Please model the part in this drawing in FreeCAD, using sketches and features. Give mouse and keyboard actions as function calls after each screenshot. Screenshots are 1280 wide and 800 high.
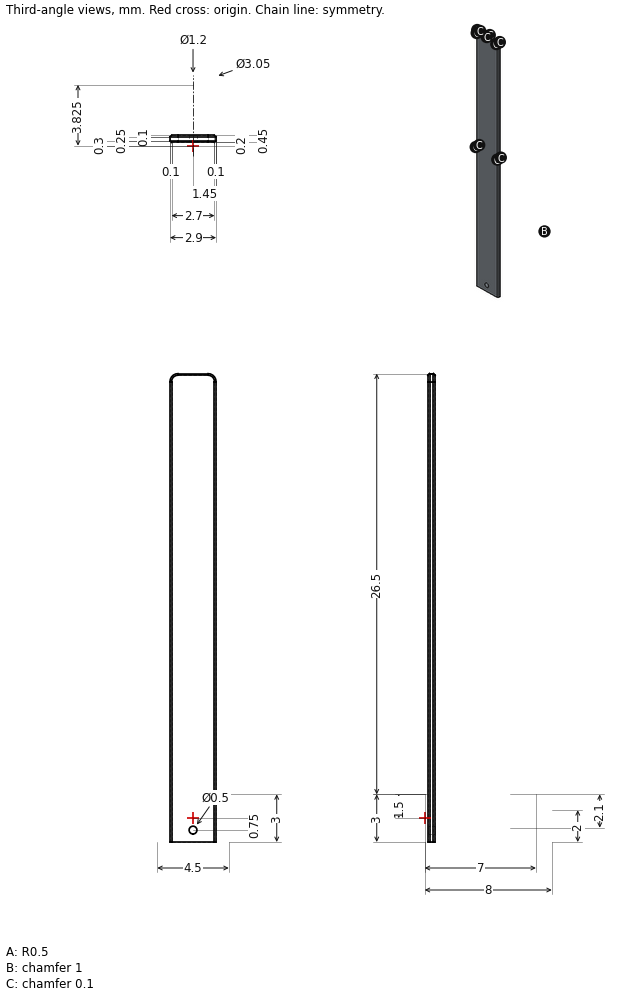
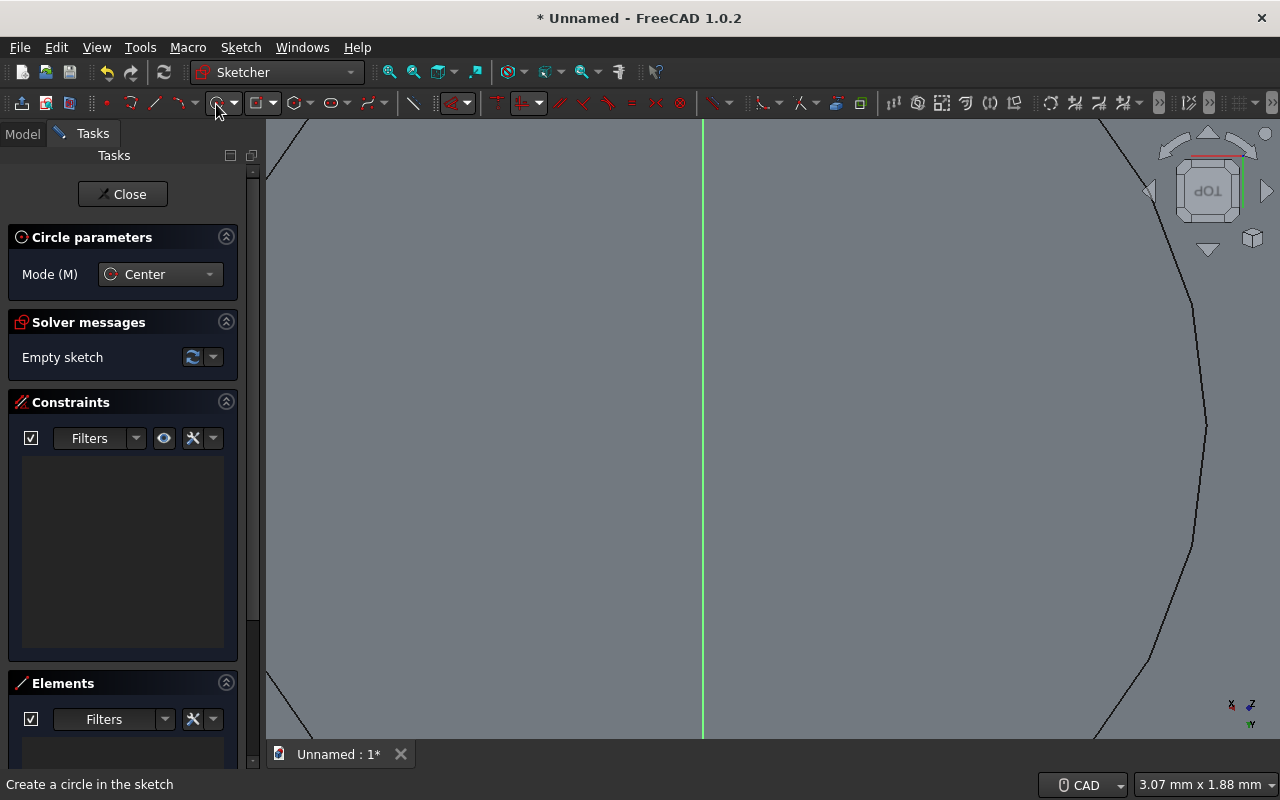
click(703, 425)
click(843, 285)
key(Escape)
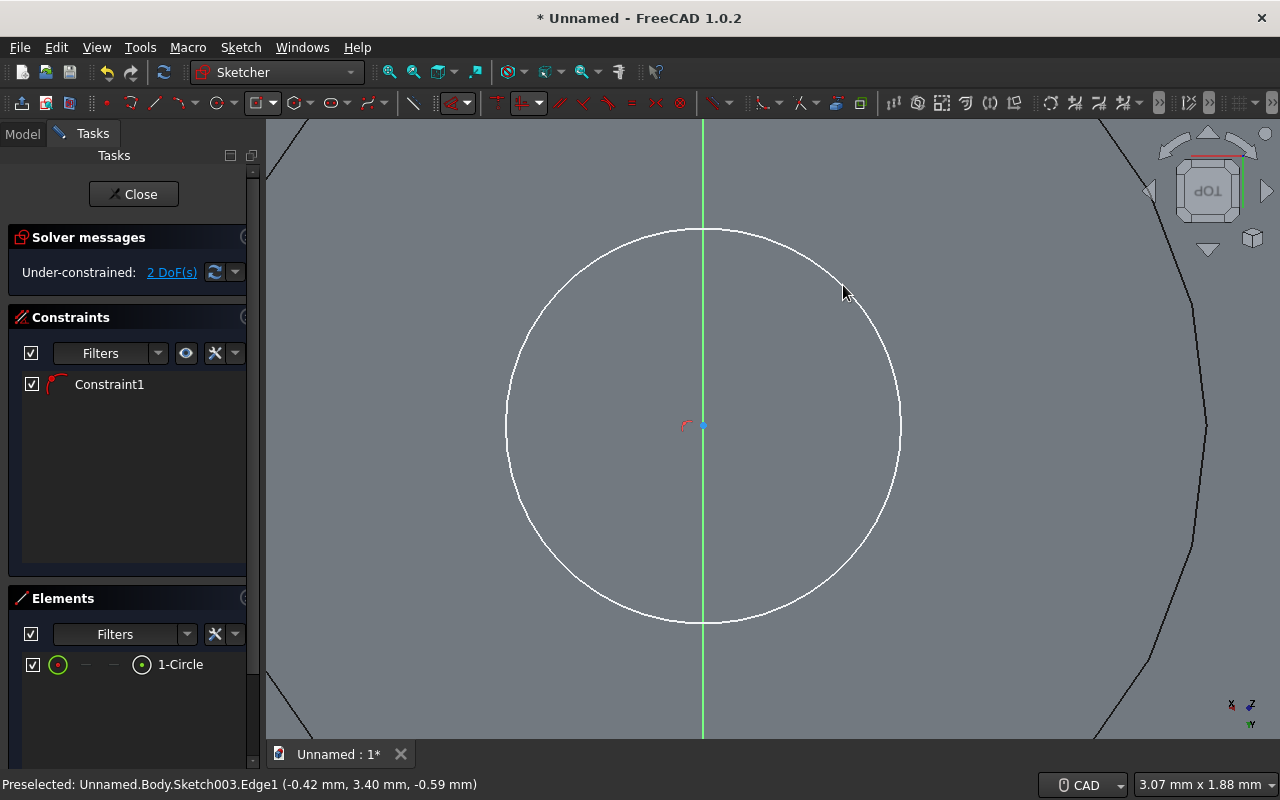
key(d)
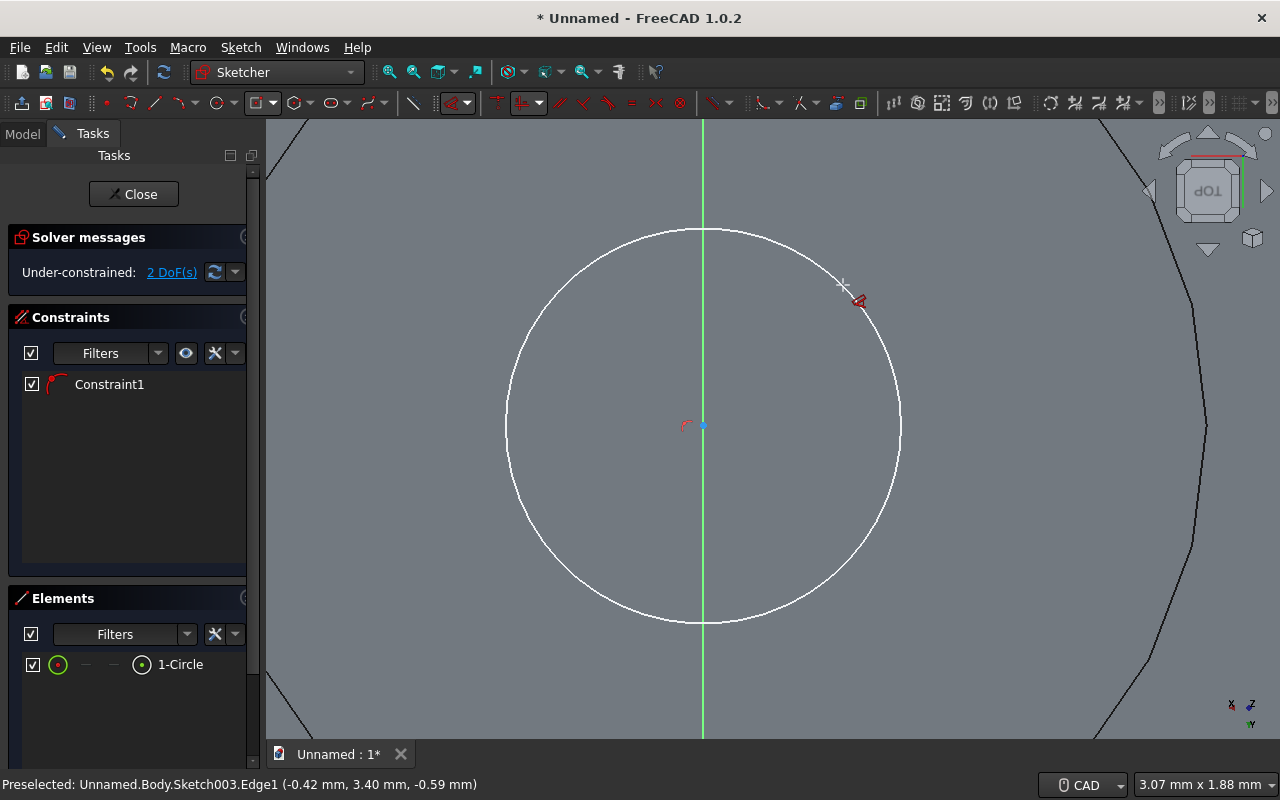
click(843, 286)
click(866, 263)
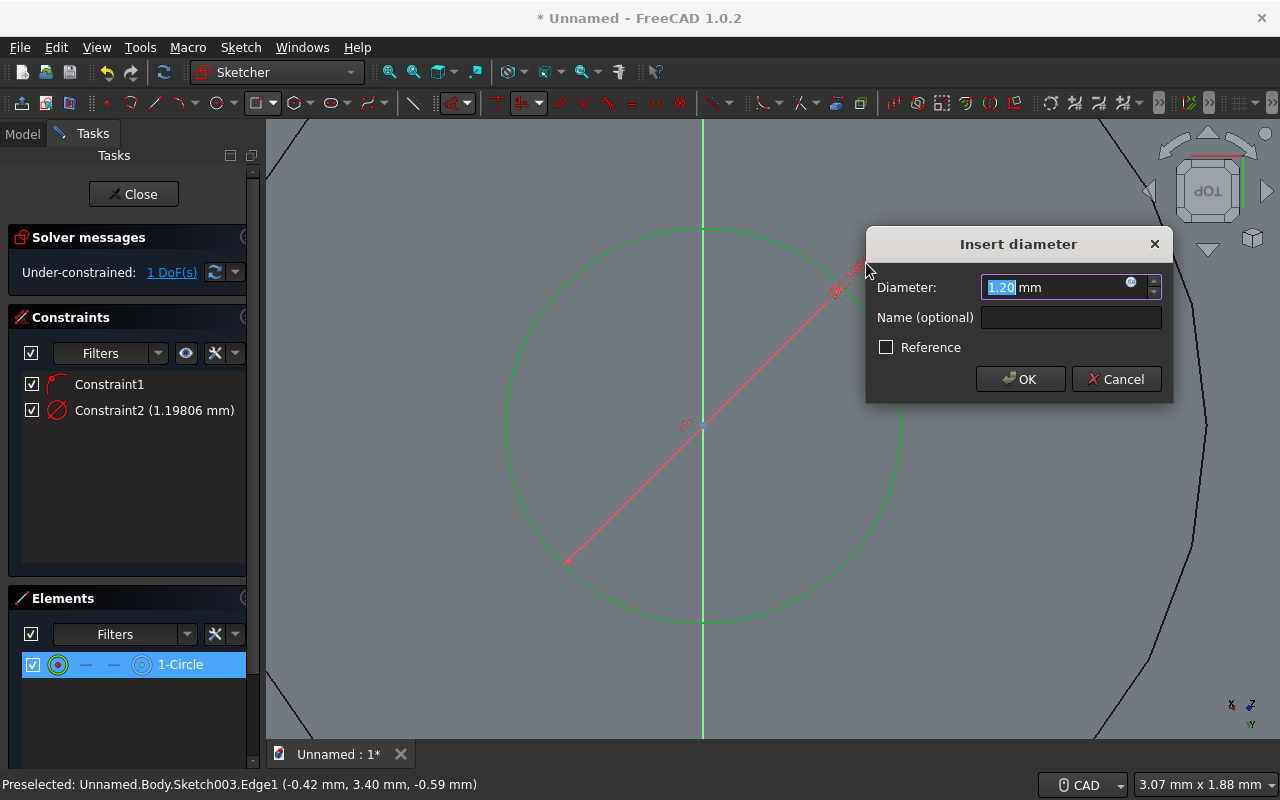
text(1.2)
key(Return)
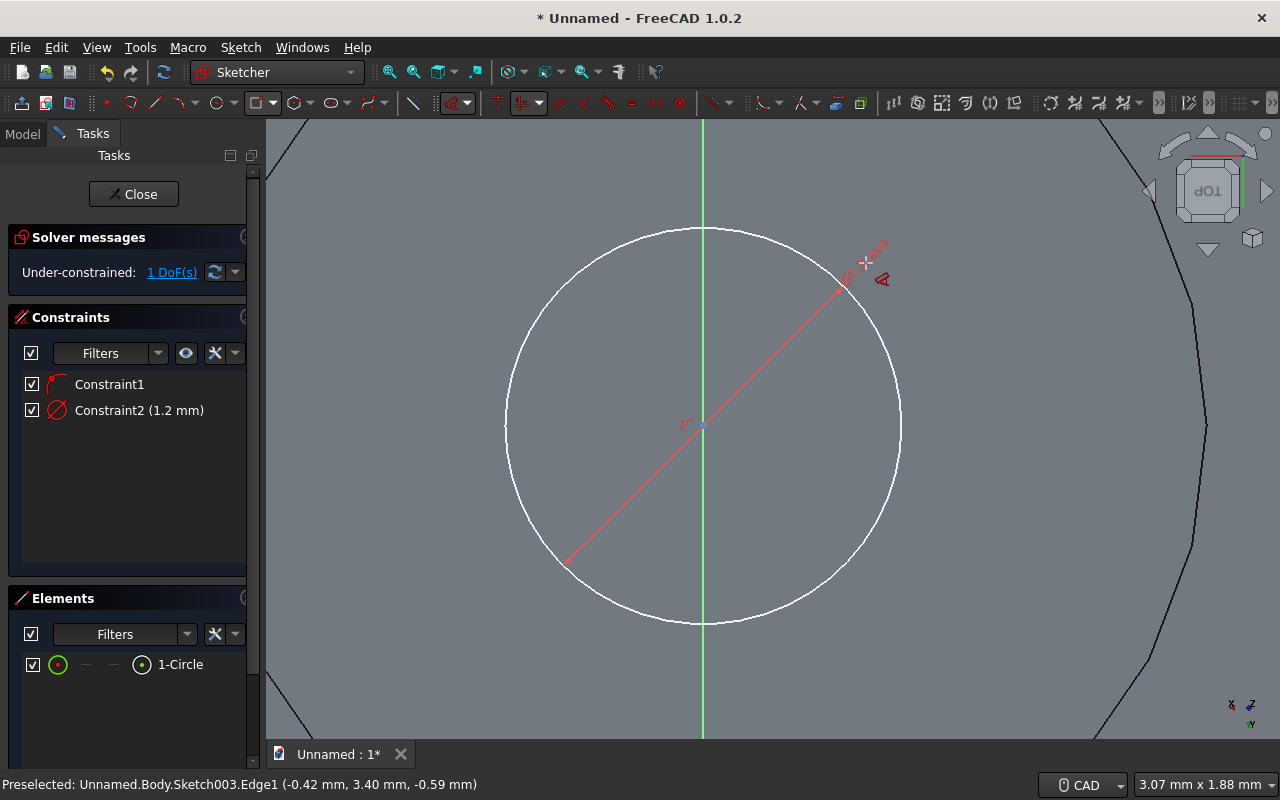
click(703, 426)
click(737, 286)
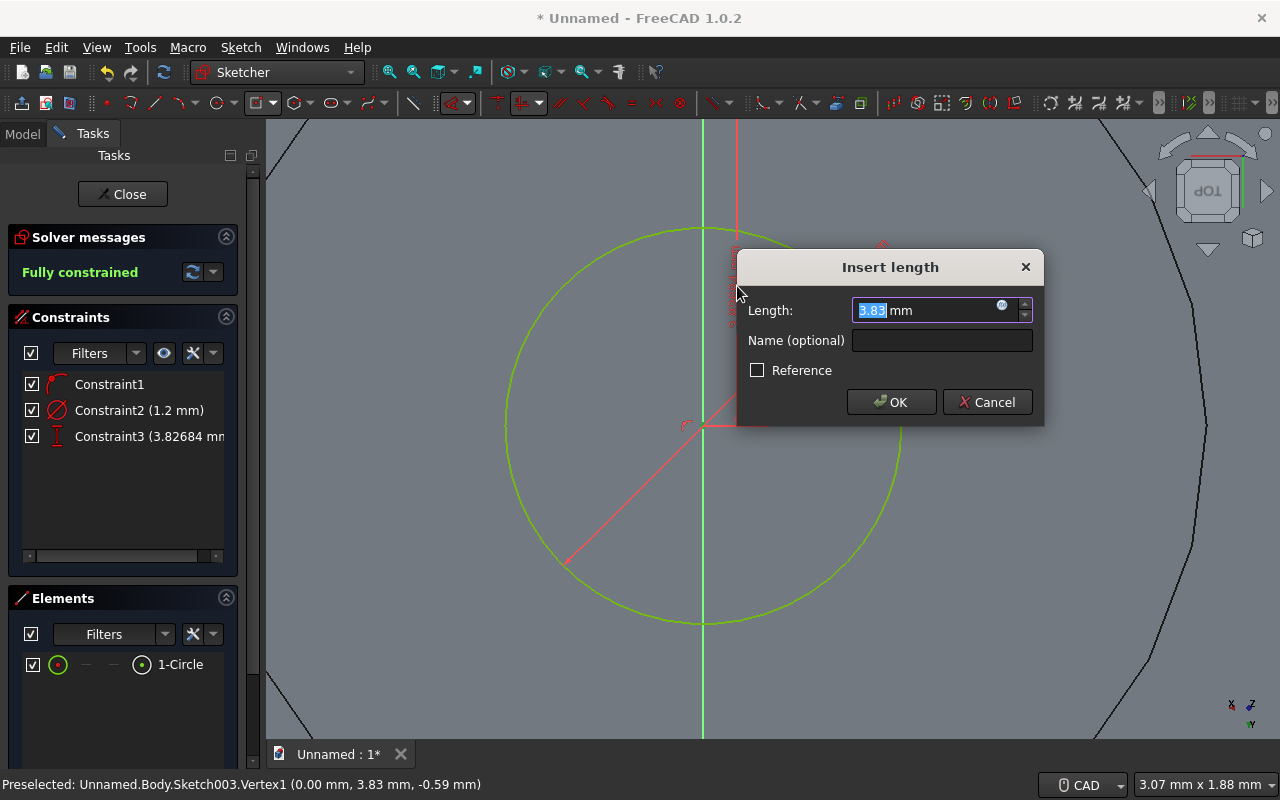
text(3.825)
key(Return)
key(Escape)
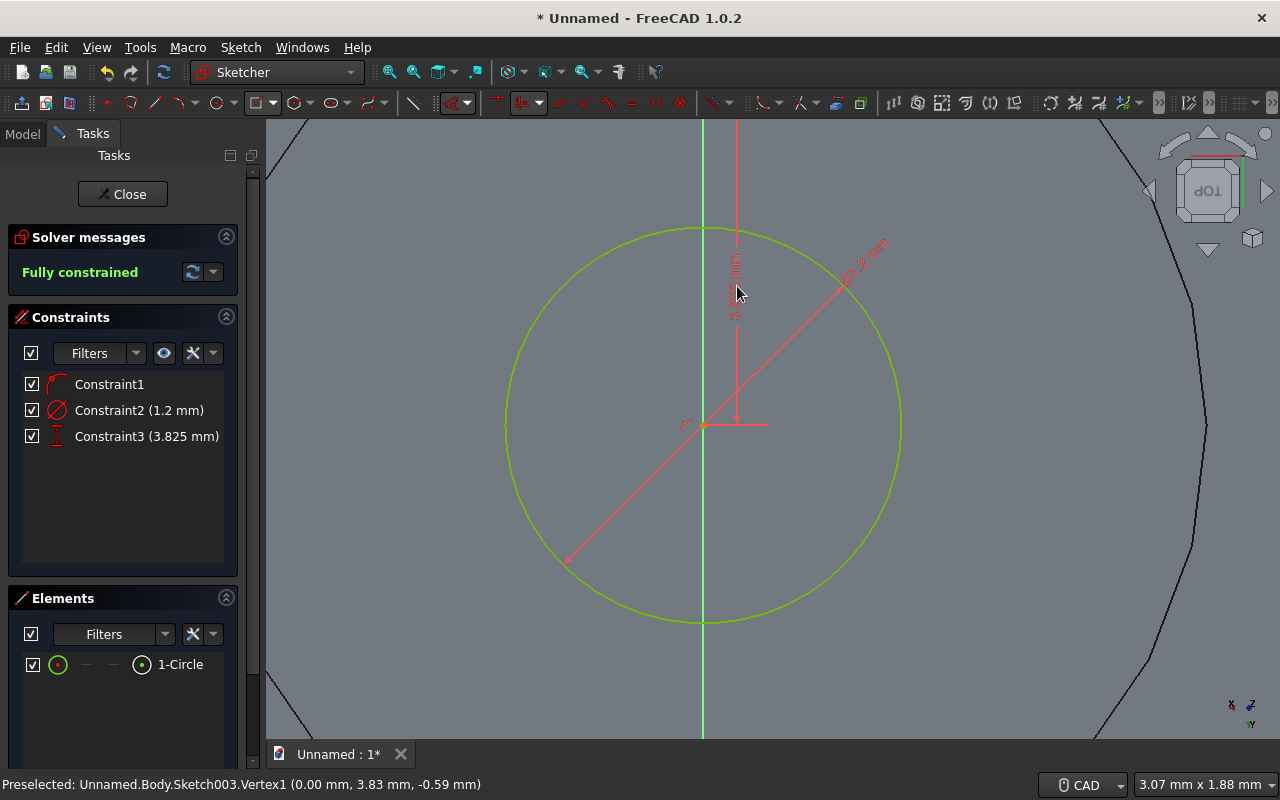
click(123, 194)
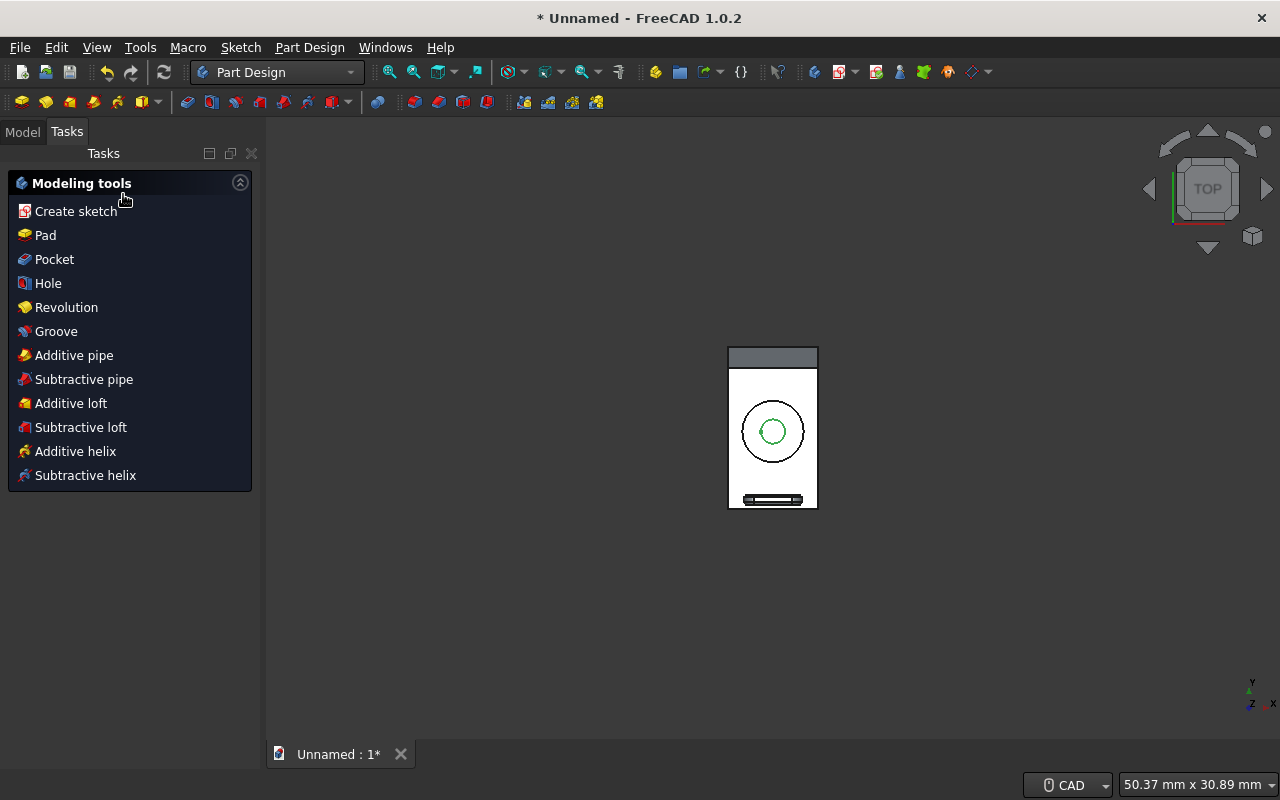
click(188, 102)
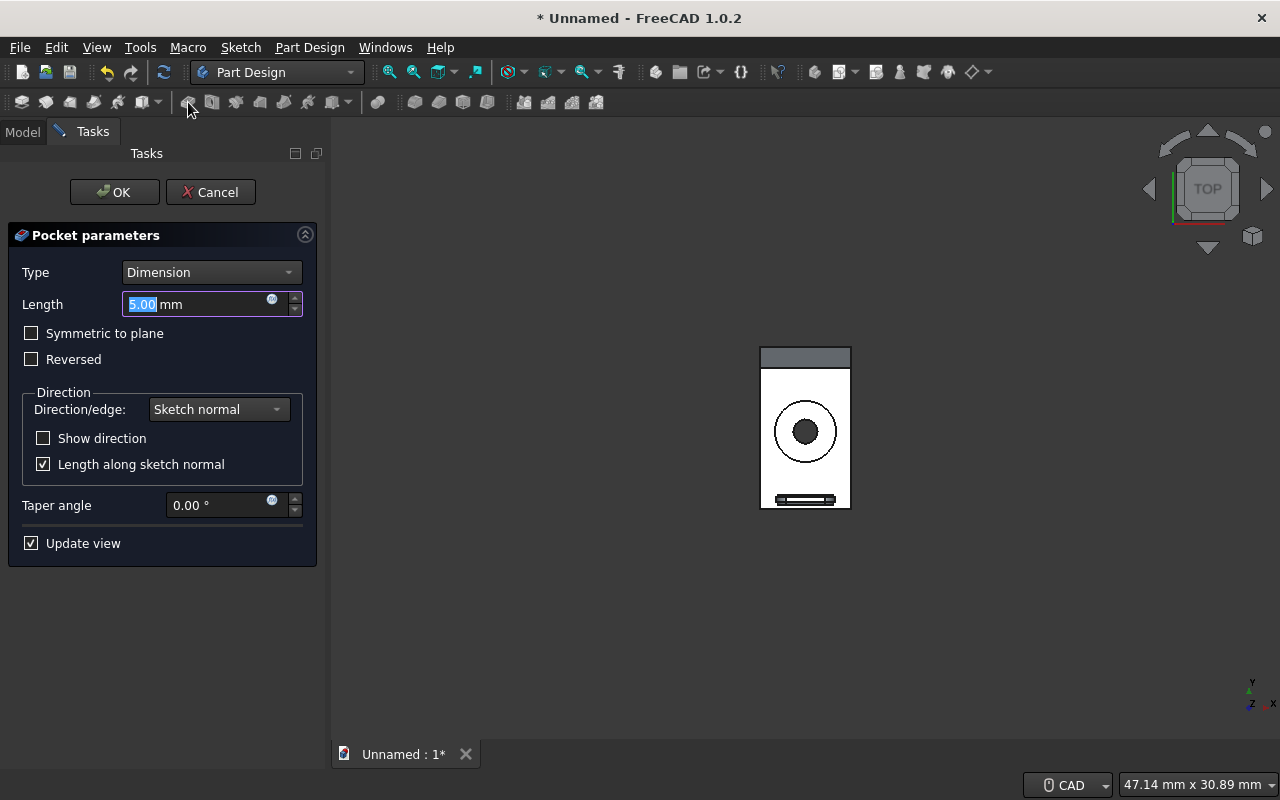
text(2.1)
key(Tab)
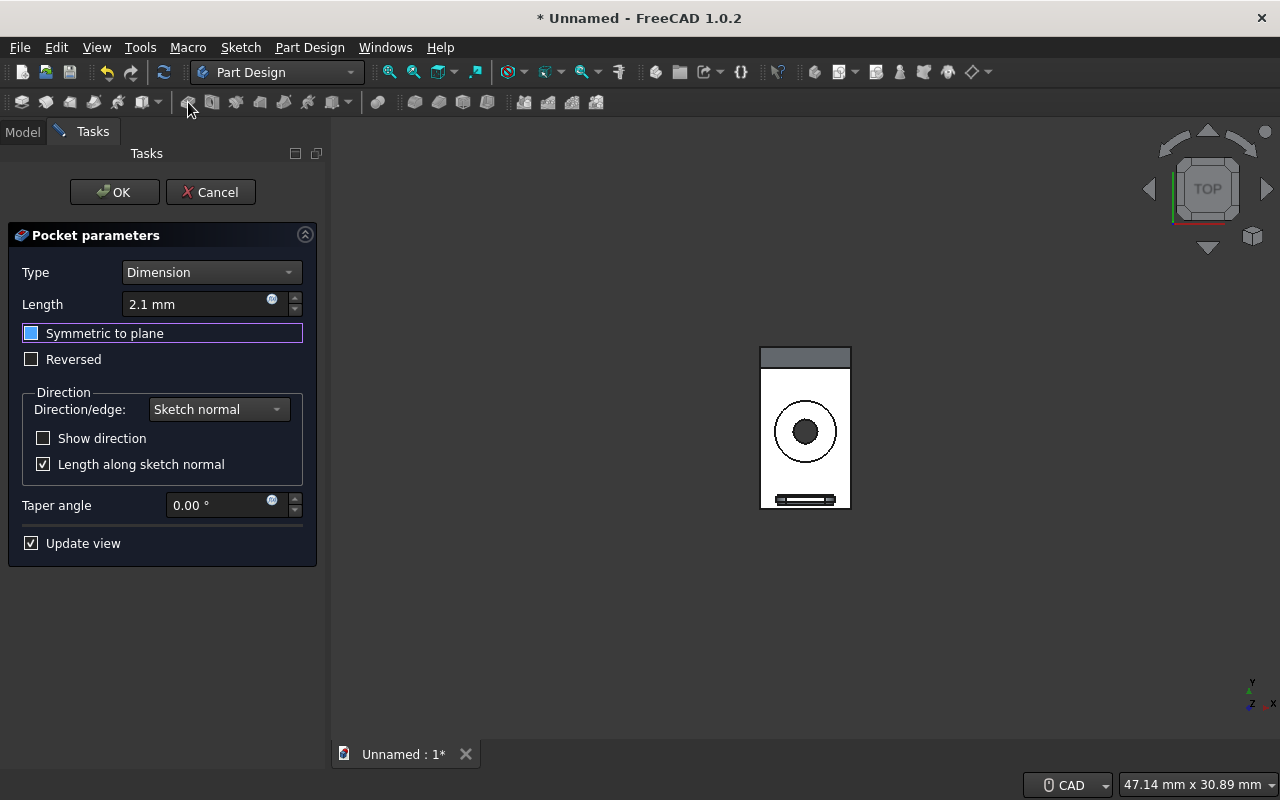
click(115, 192)